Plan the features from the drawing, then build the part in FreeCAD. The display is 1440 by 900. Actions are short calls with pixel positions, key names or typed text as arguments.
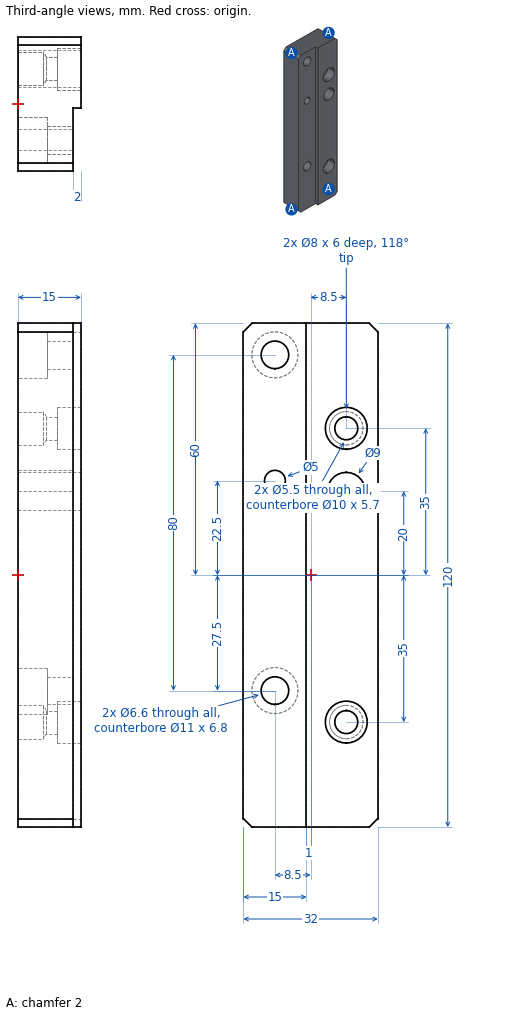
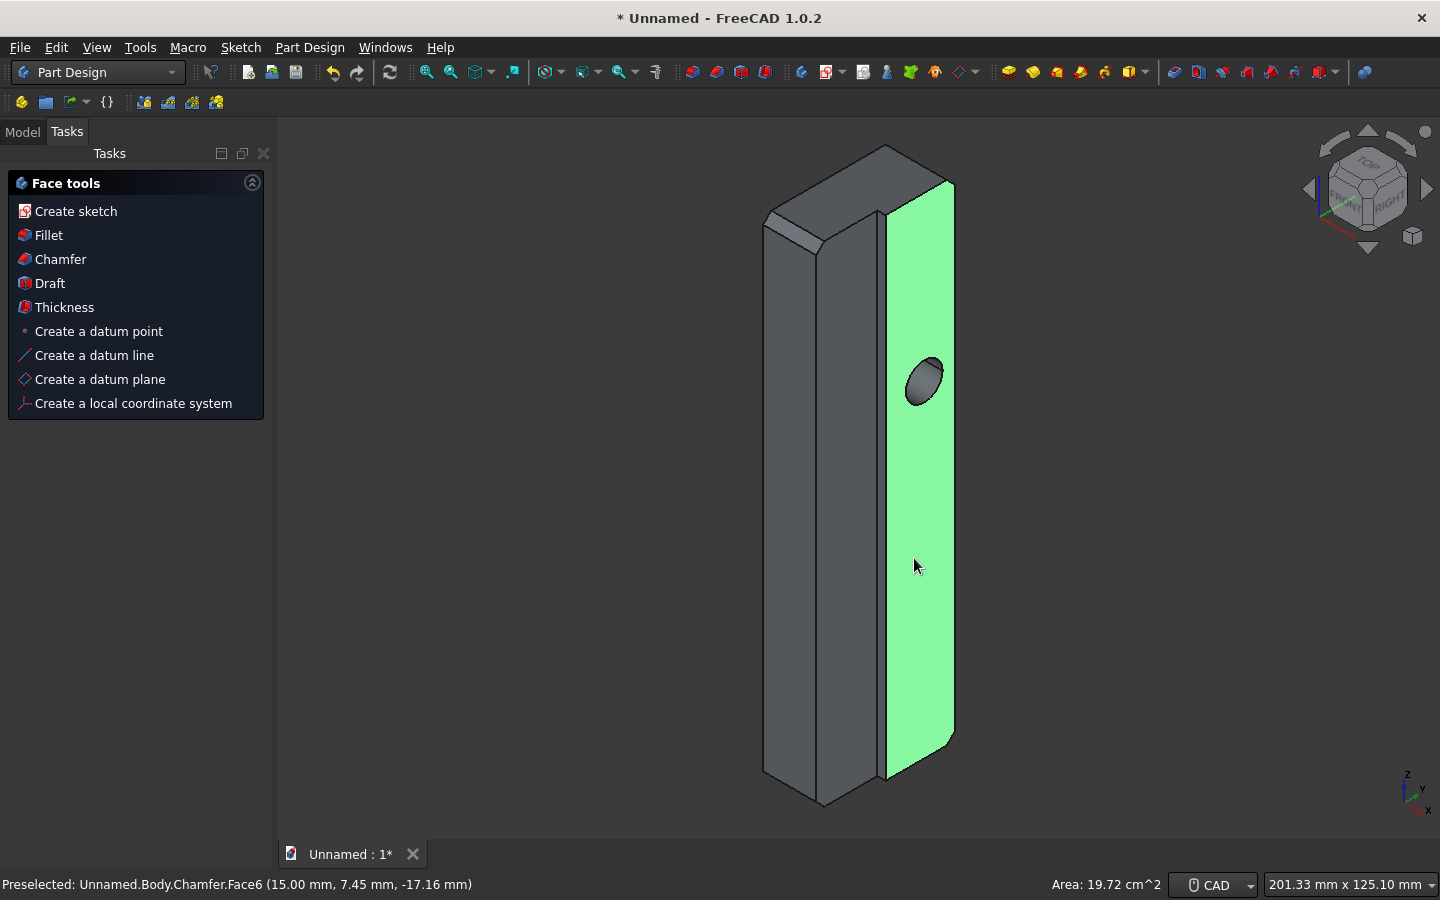
click(826, 72)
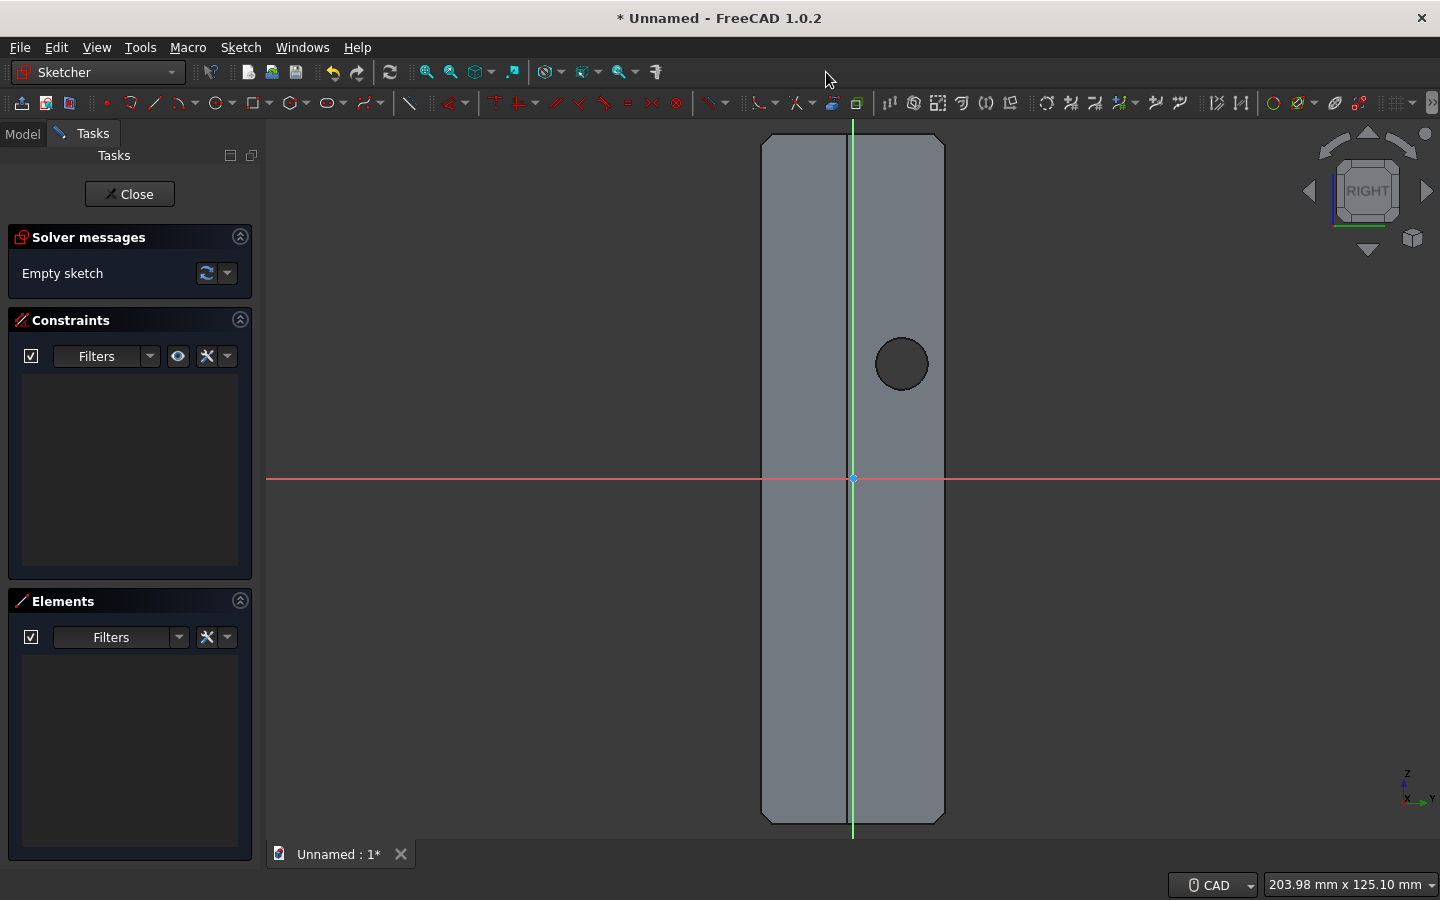
click(216, 104)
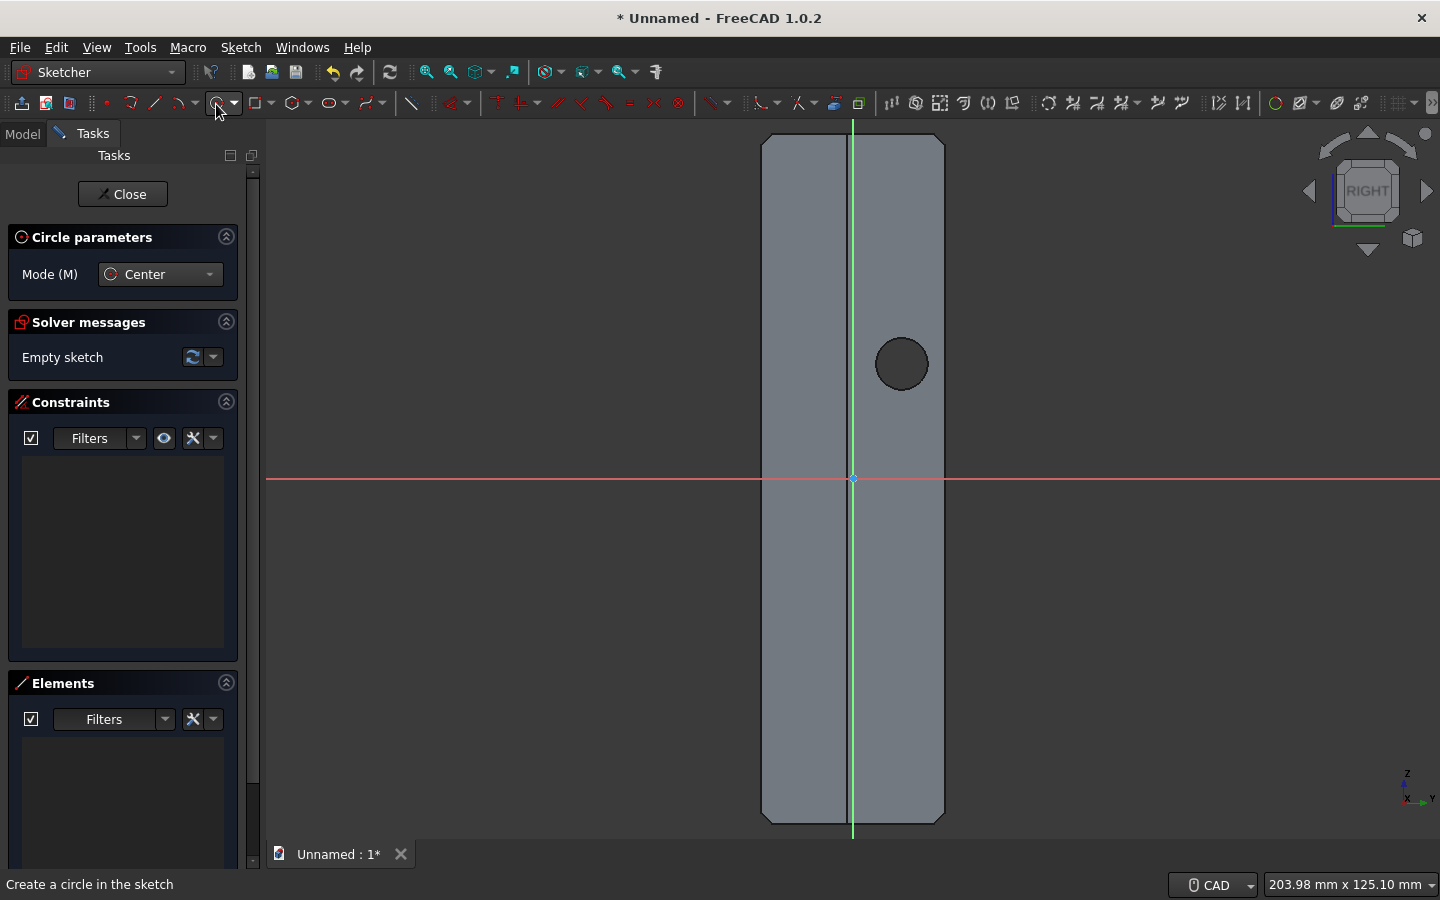
scroll(902, 278, up, 2)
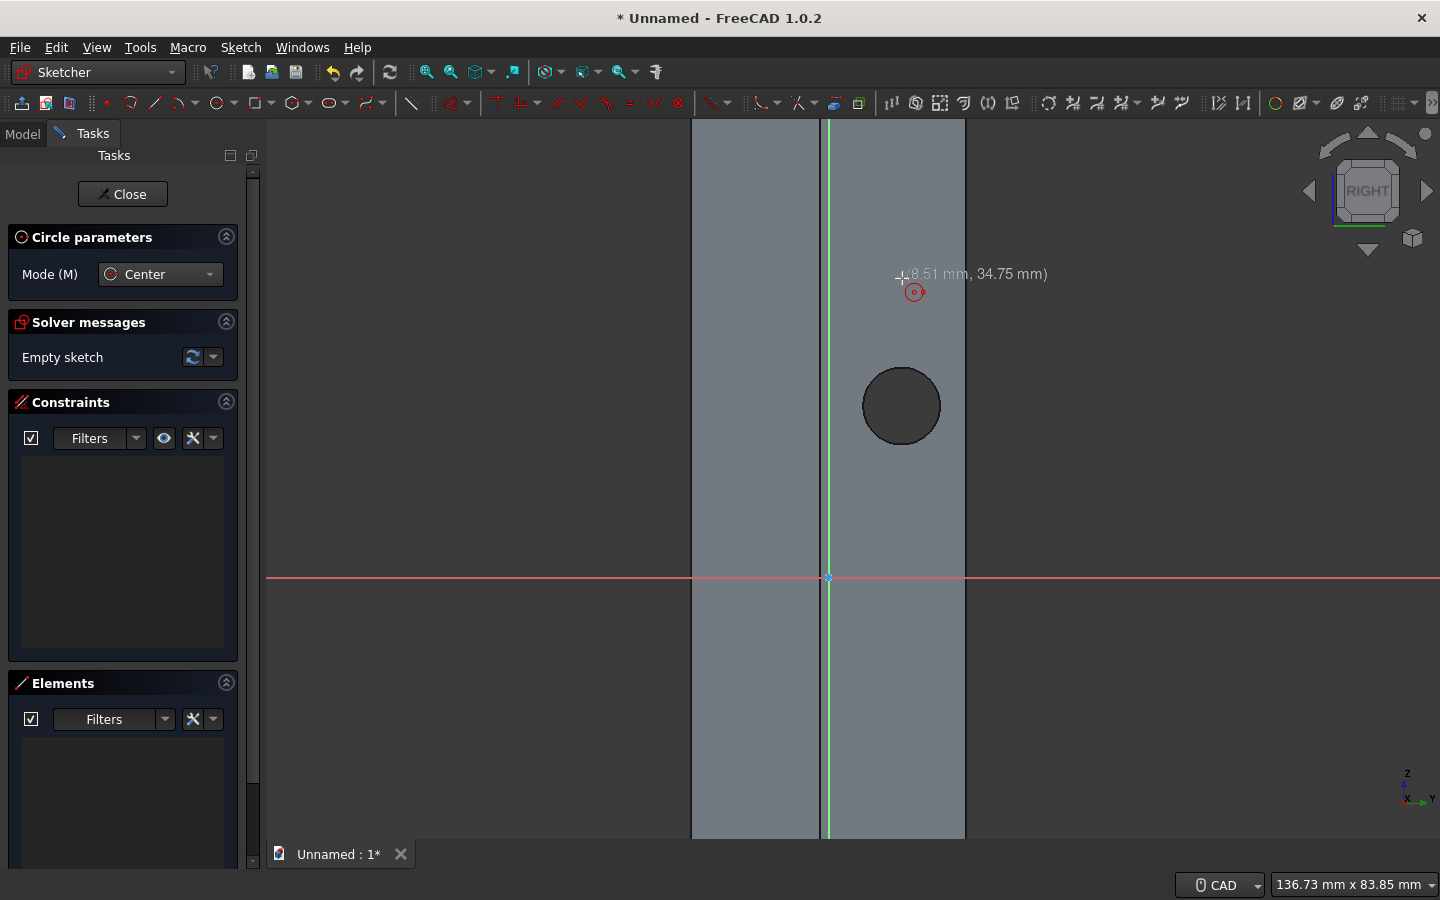
click(902, 277)
click(918, 261)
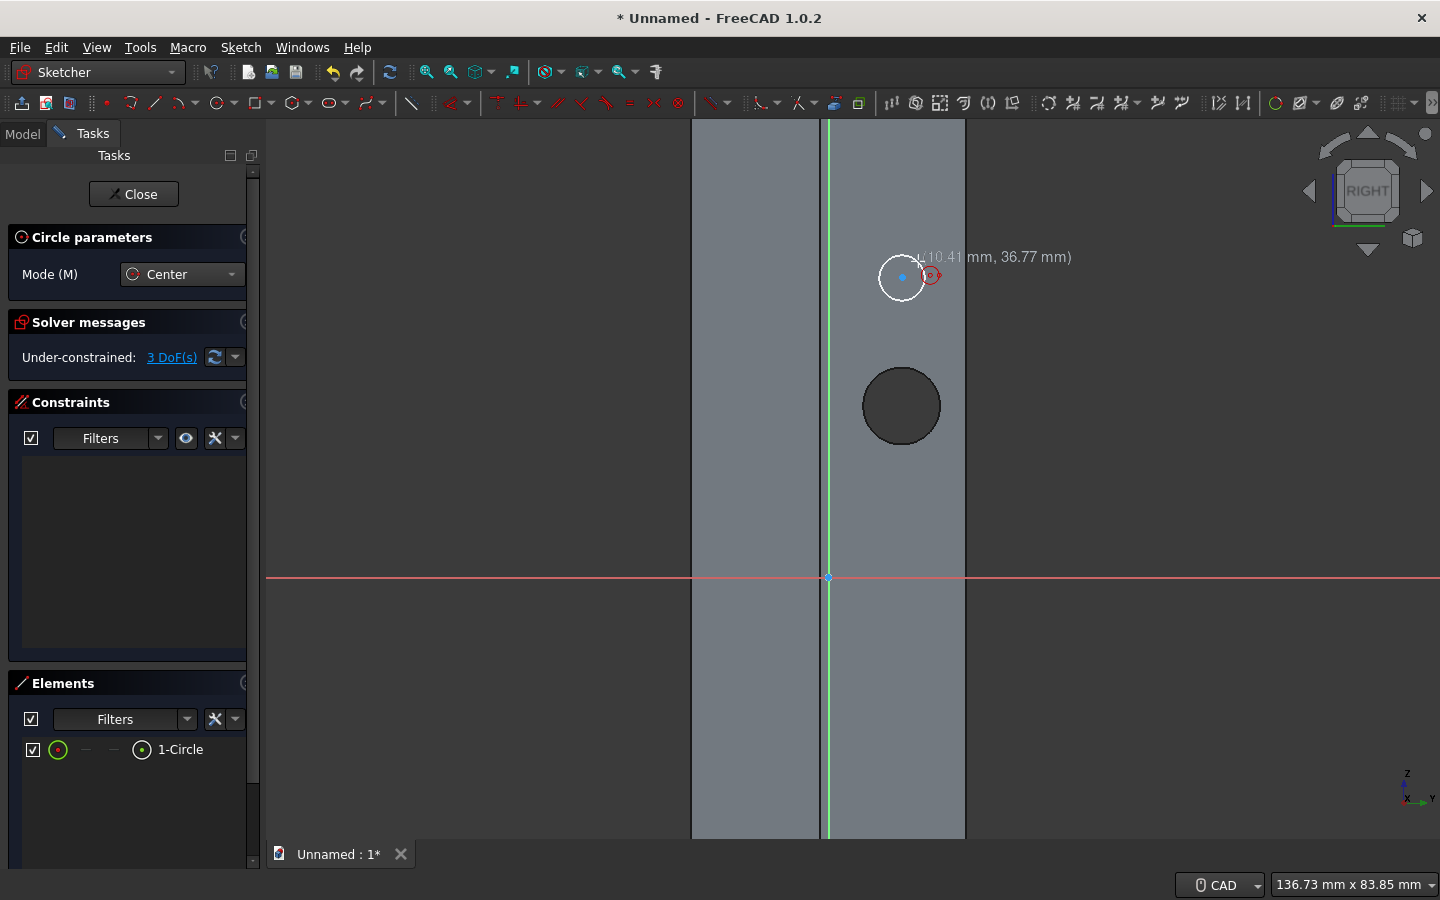
scroll(597, 278, down, 2)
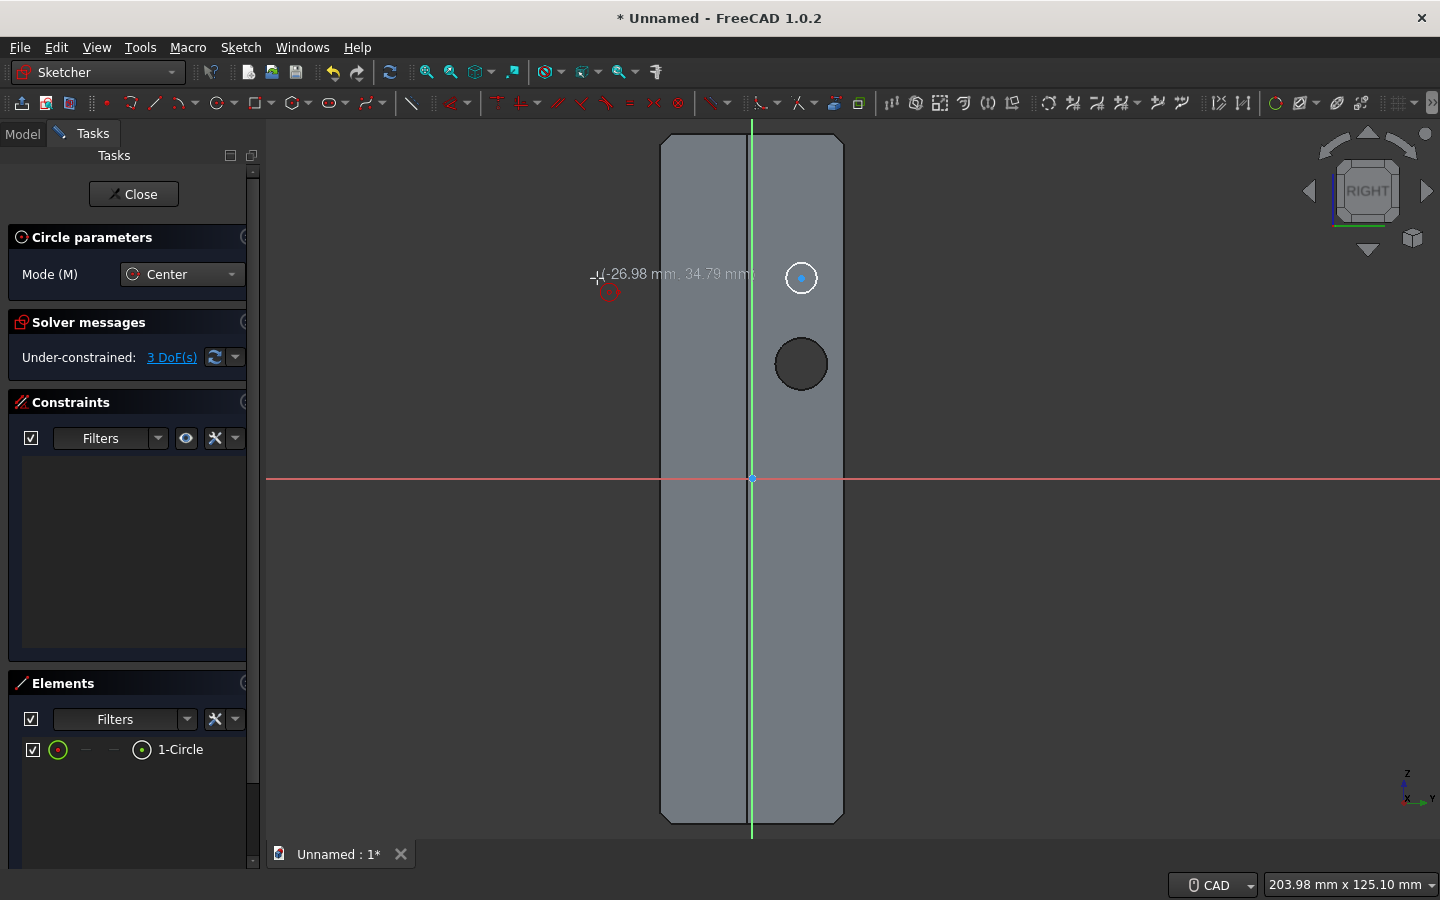
scroll(801, 680, up, 2)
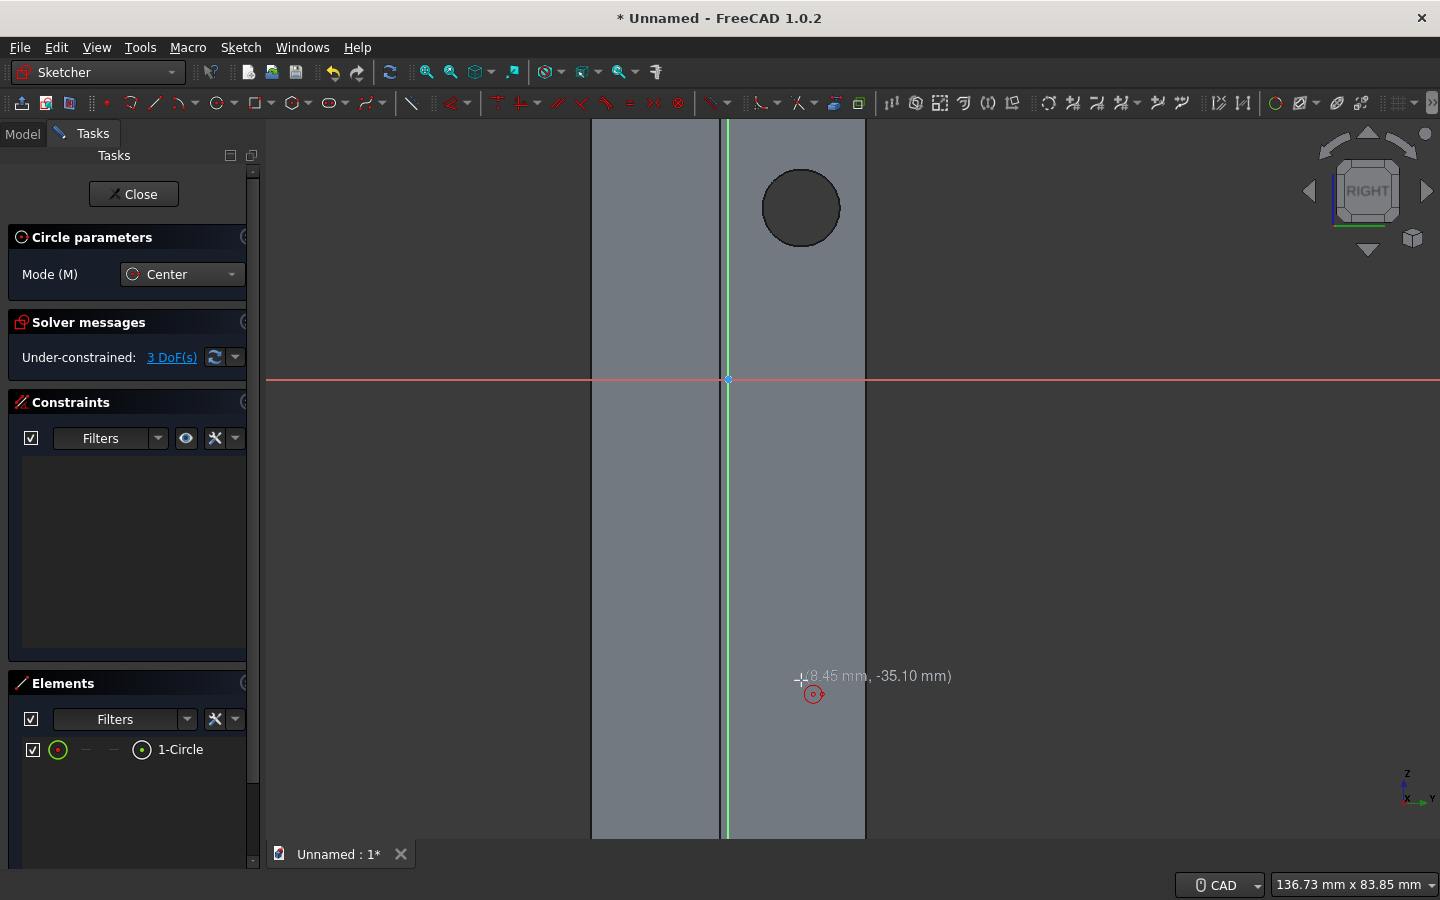
click(801, 680)
click(818, 664)
key(Escape)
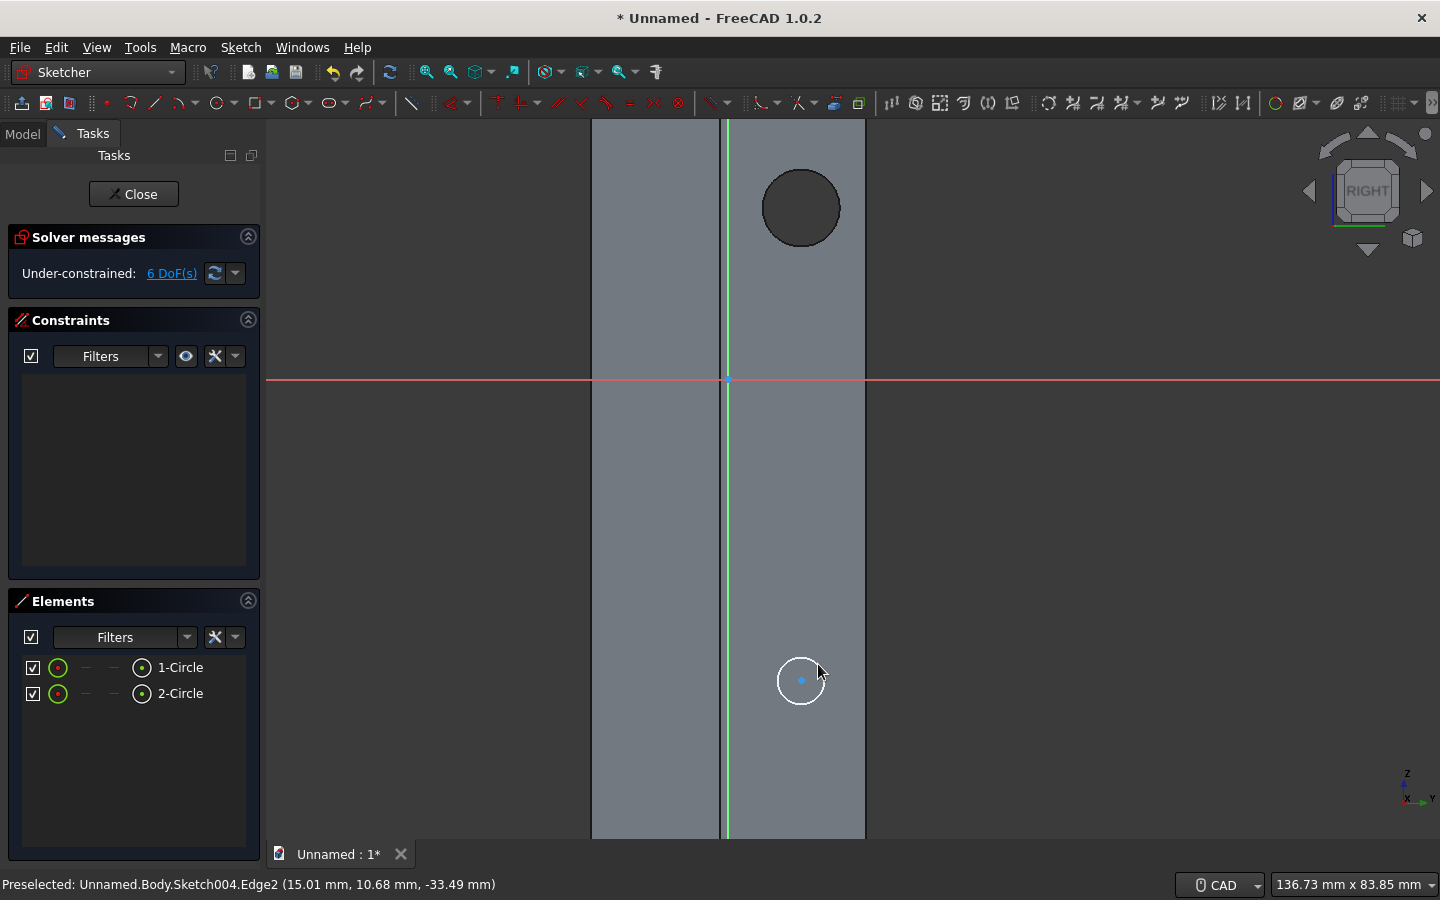
scroll(801, 681, down, 2)